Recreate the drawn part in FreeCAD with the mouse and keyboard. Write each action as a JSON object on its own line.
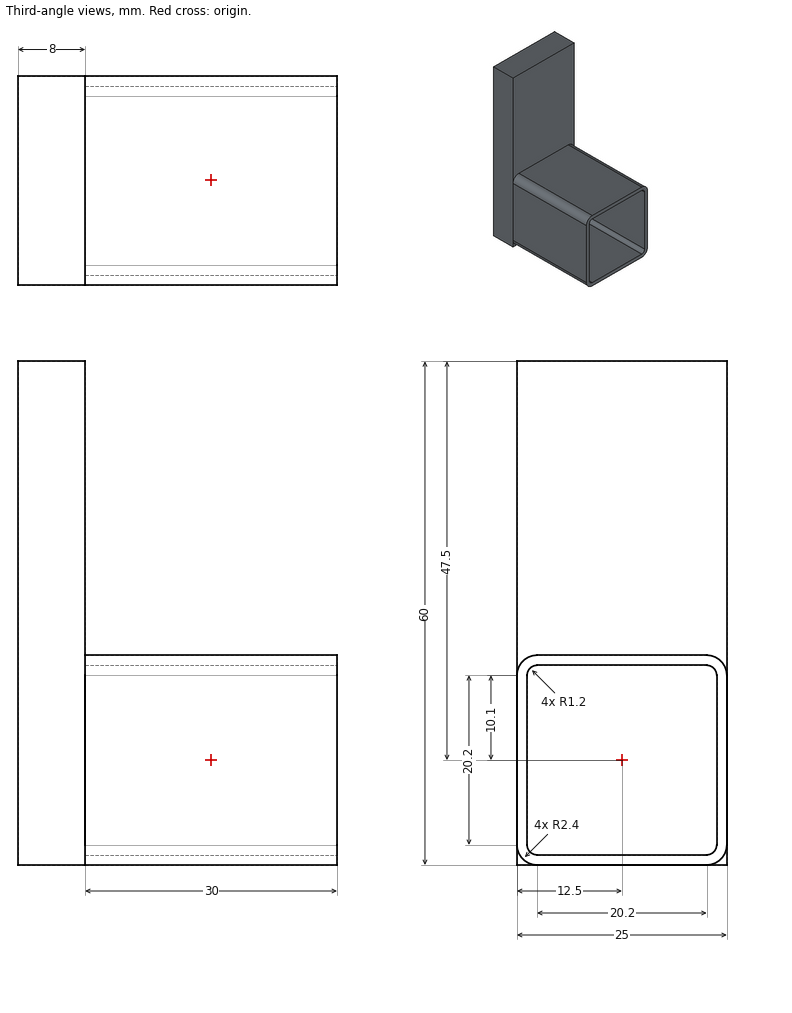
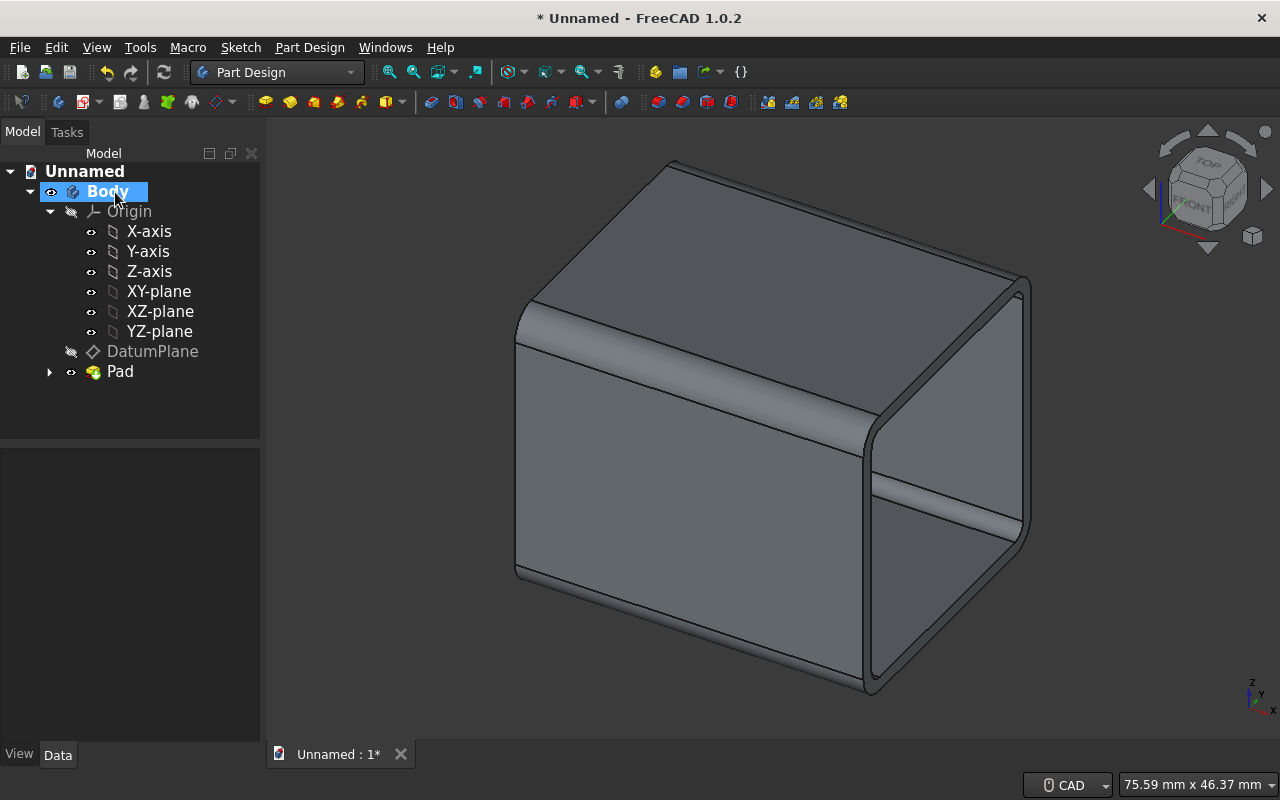
{"action": "left_click", "coordinate": [60, 102]}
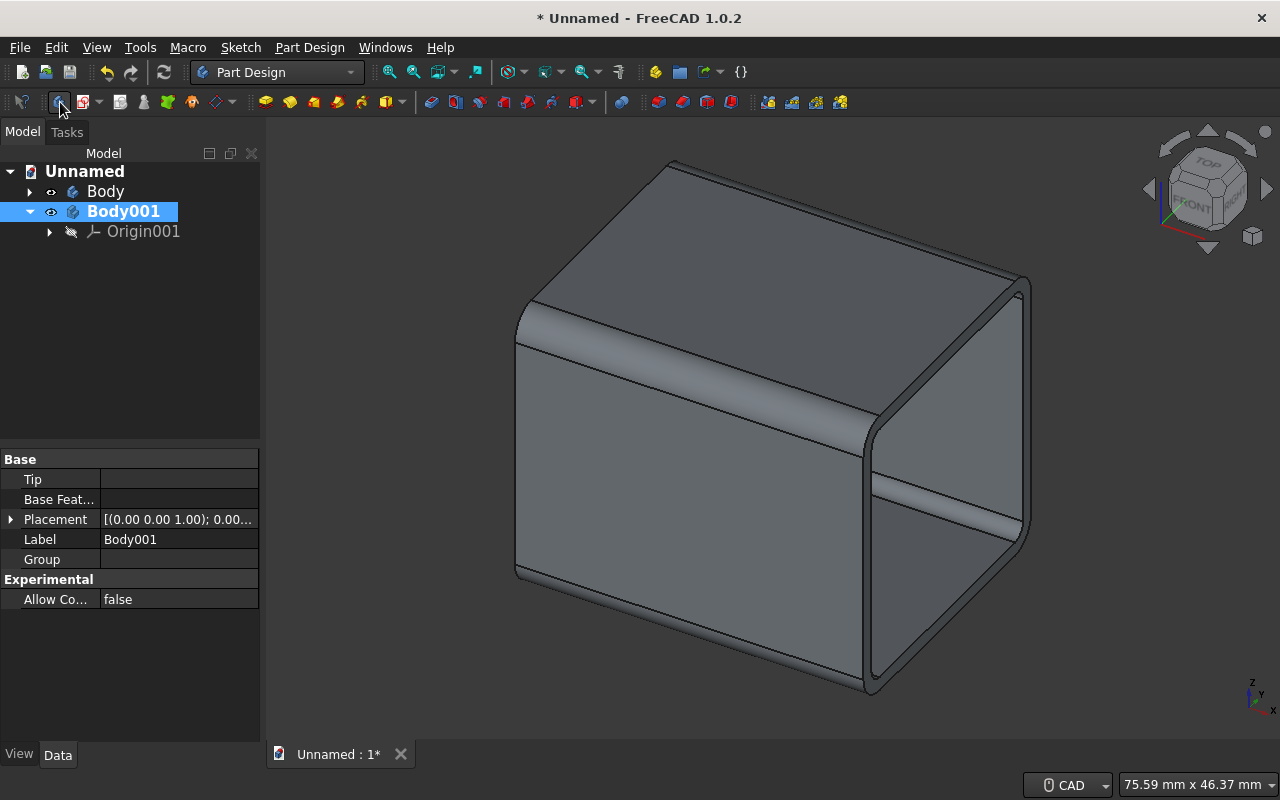
{"action": "left_click", "coordinate": [50, 232]}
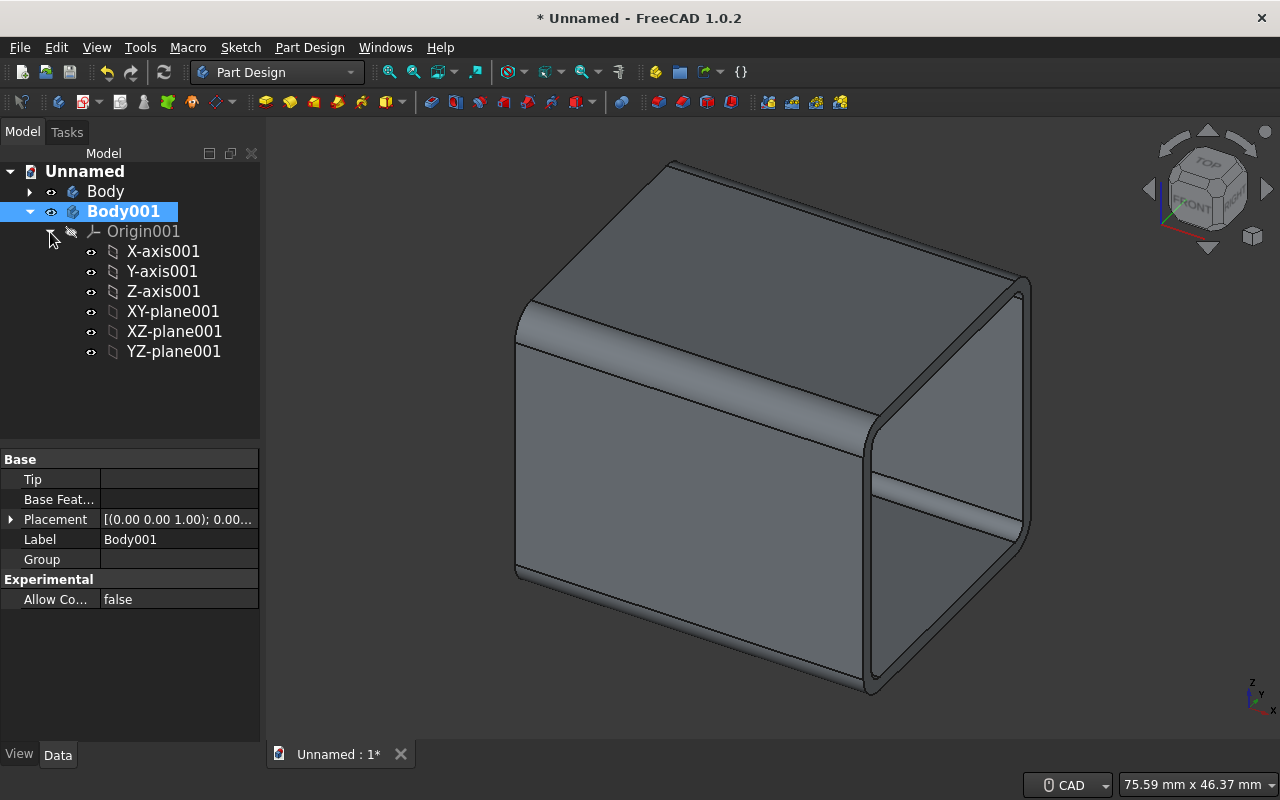
{"action": "left_click", "coordinate": [136, 352]}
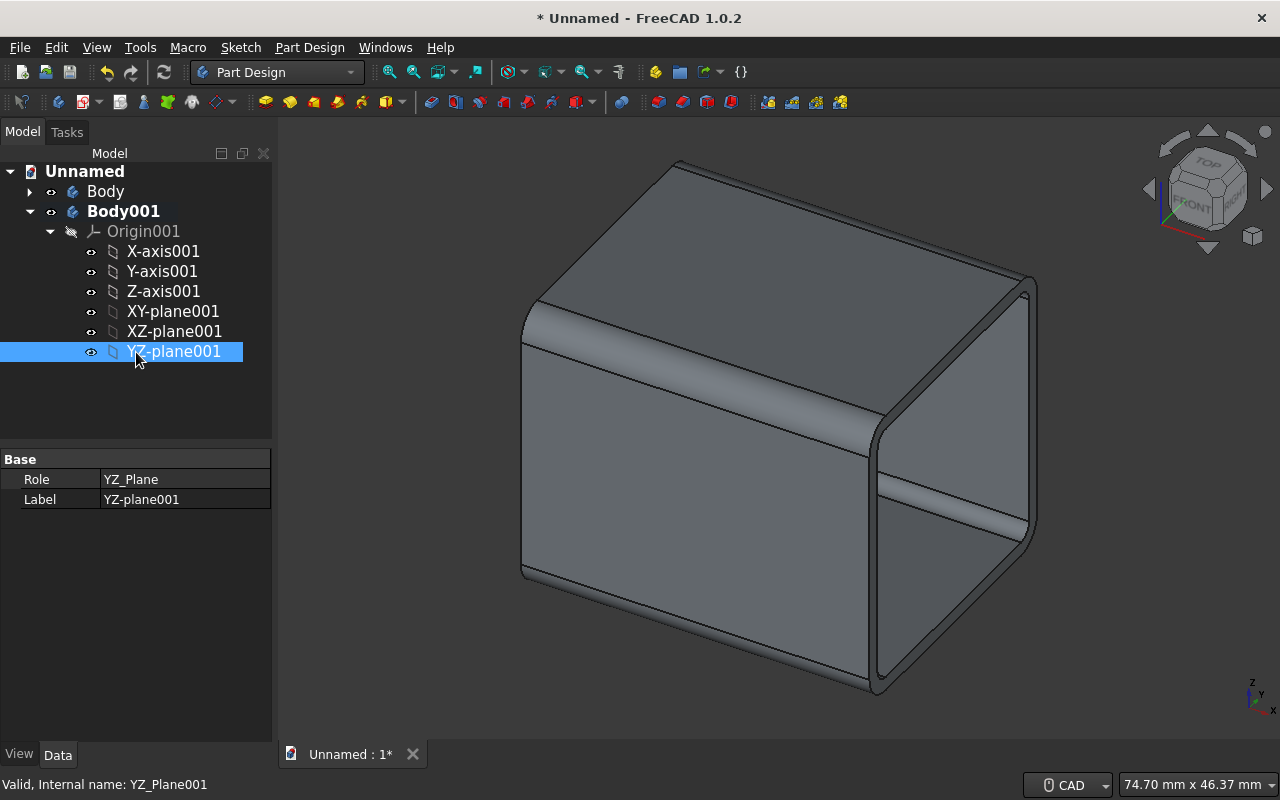
{"action": "left_click", "coordinate": [216, 102]}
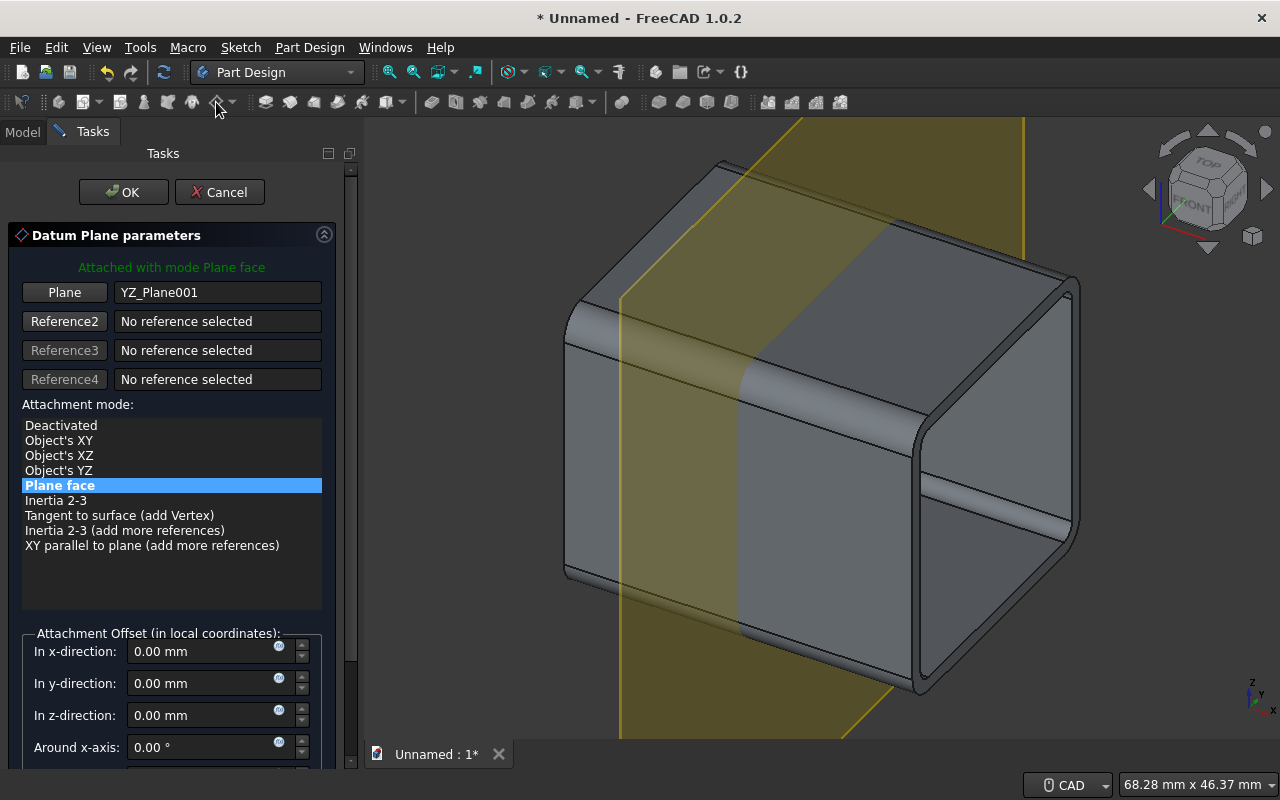
{"action": "triple_click", "coordinate": [210, 715]}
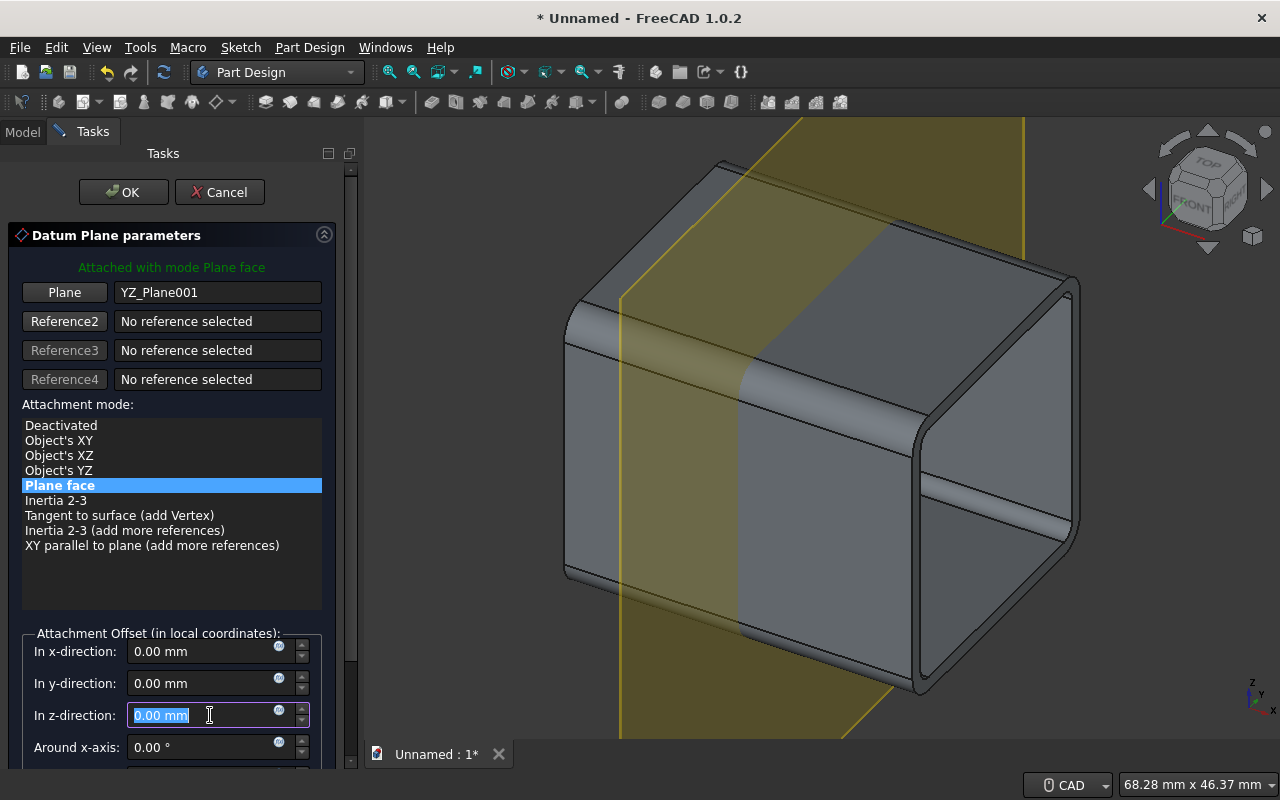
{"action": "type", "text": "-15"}
{"action": "key", "text": "Tab"}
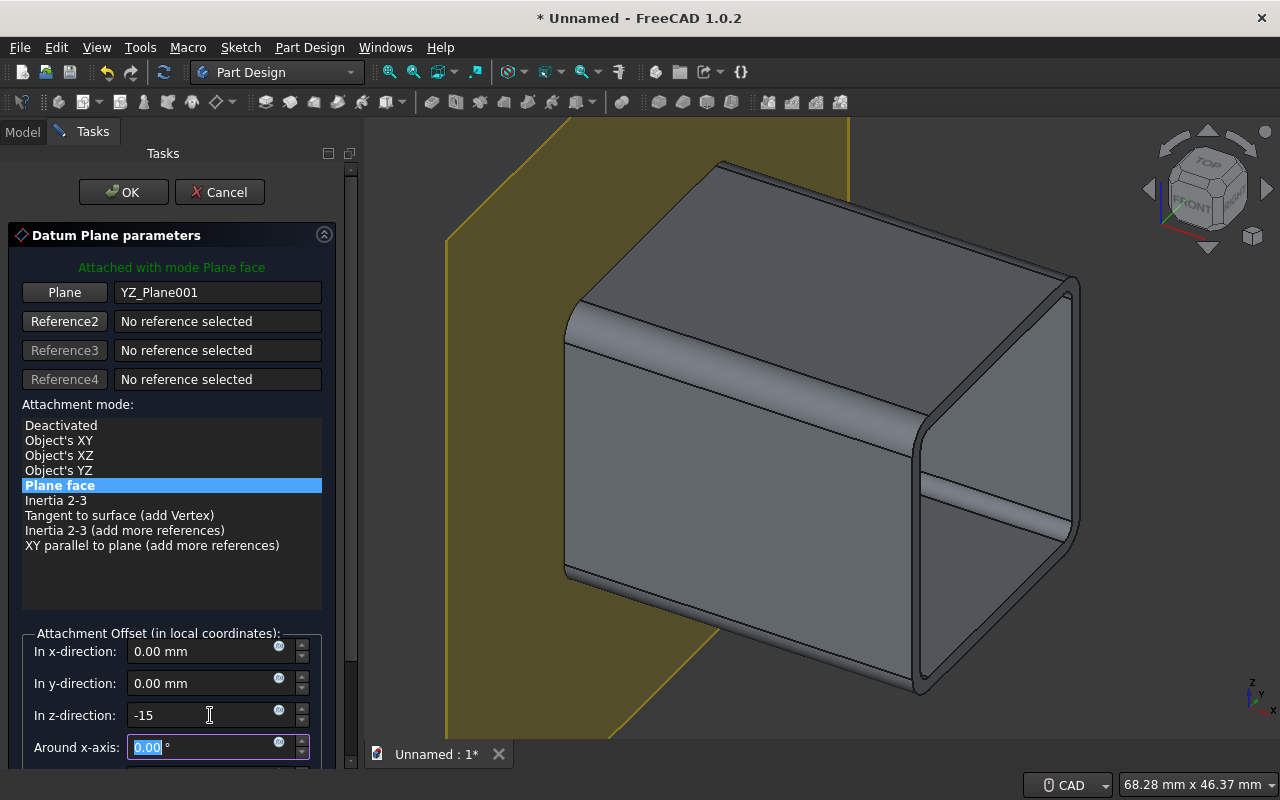
{"action": "left_click", "coordinate": [124, 192]}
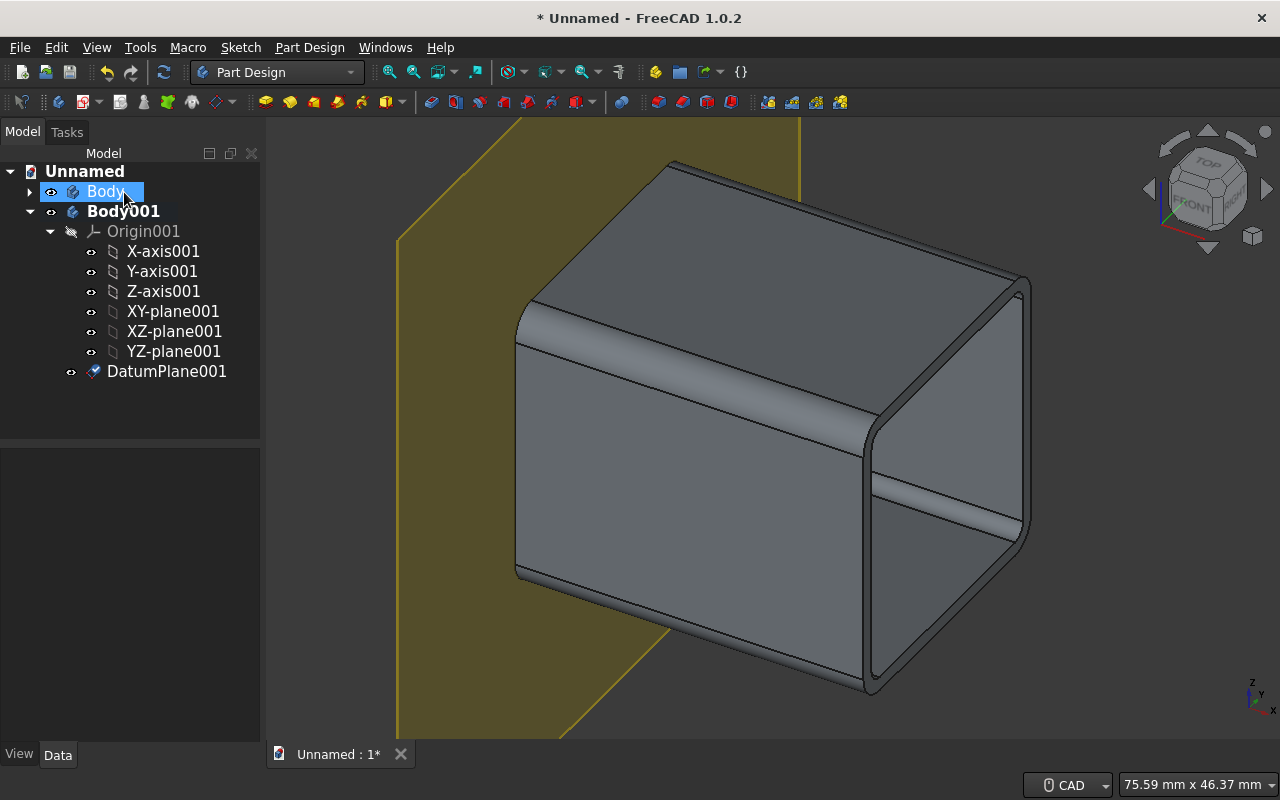
{"action": "left_click", "coordinate": [116, 372]}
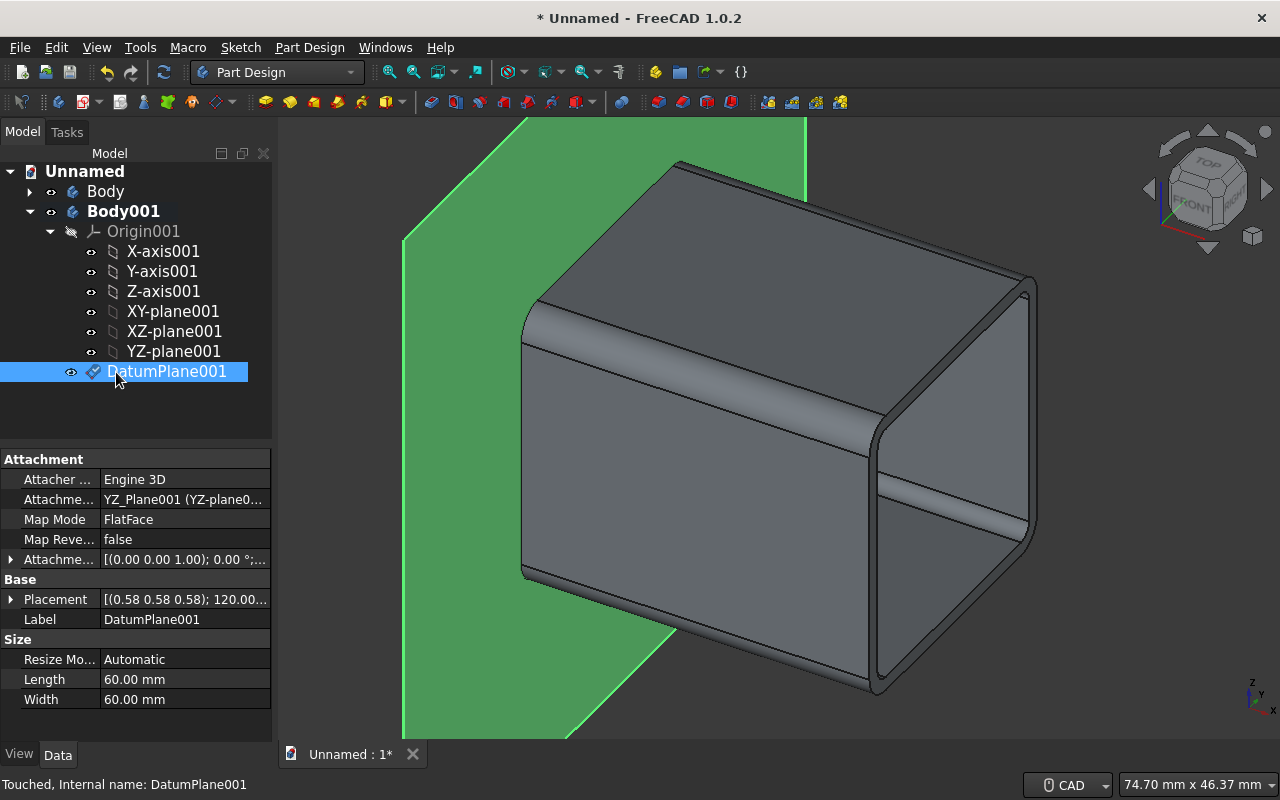
{"action": "left_click", "coordinate": [84, 102]}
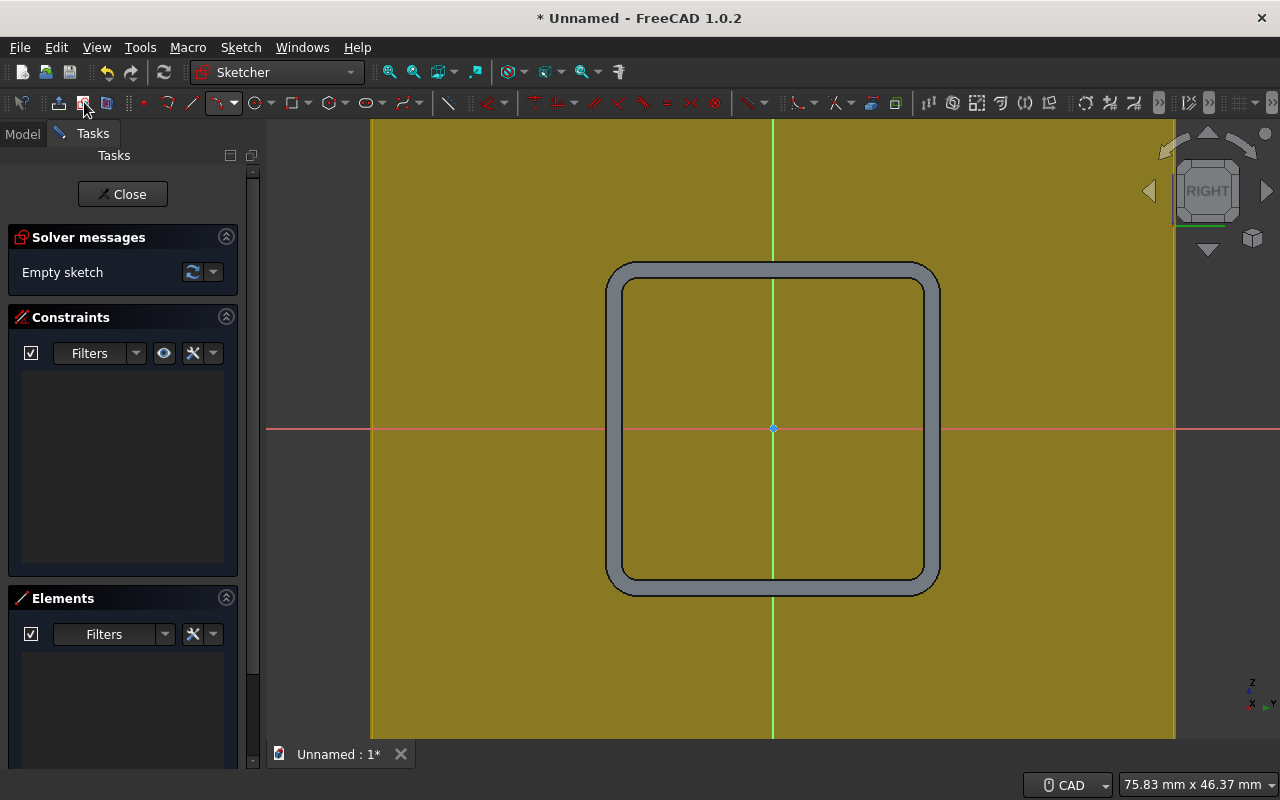
{"action": "scroll", "coordinate": [649, 620], "scroll_direction": "down", "scroll_amount": 4}